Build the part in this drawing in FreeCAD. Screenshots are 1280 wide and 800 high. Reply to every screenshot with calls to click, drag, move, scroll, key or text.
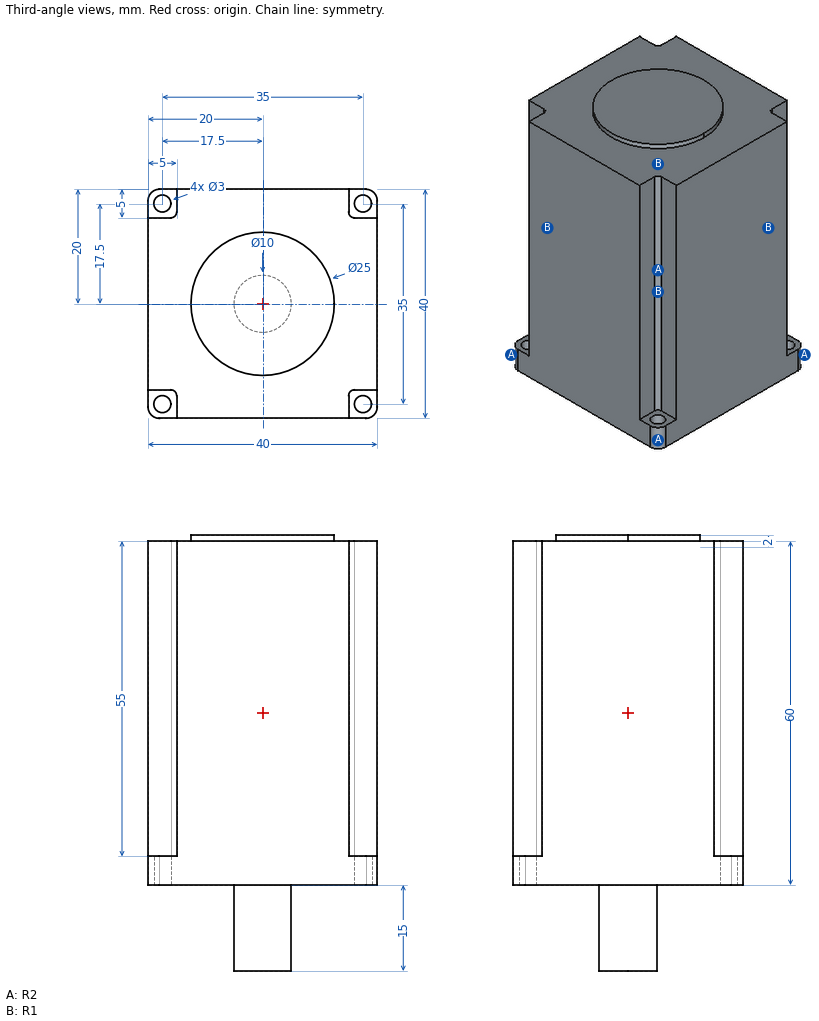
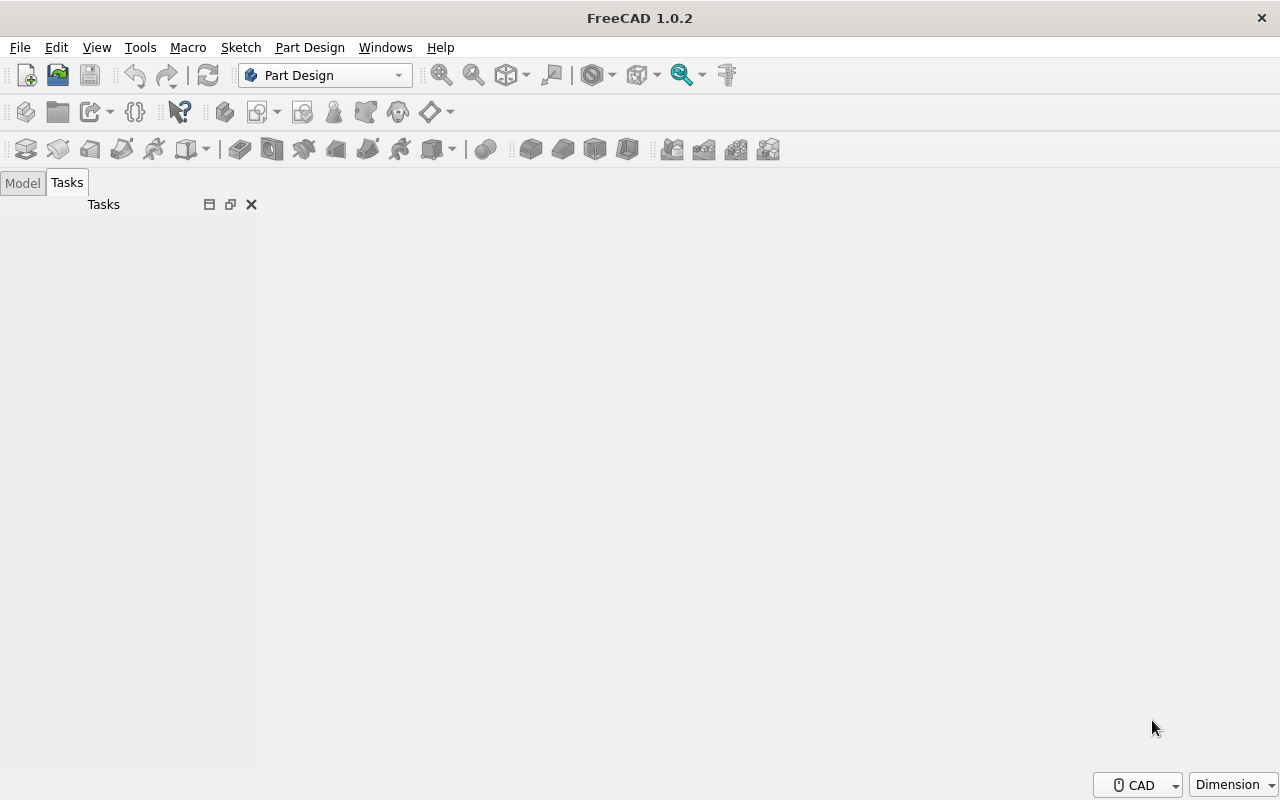
click(26, 76)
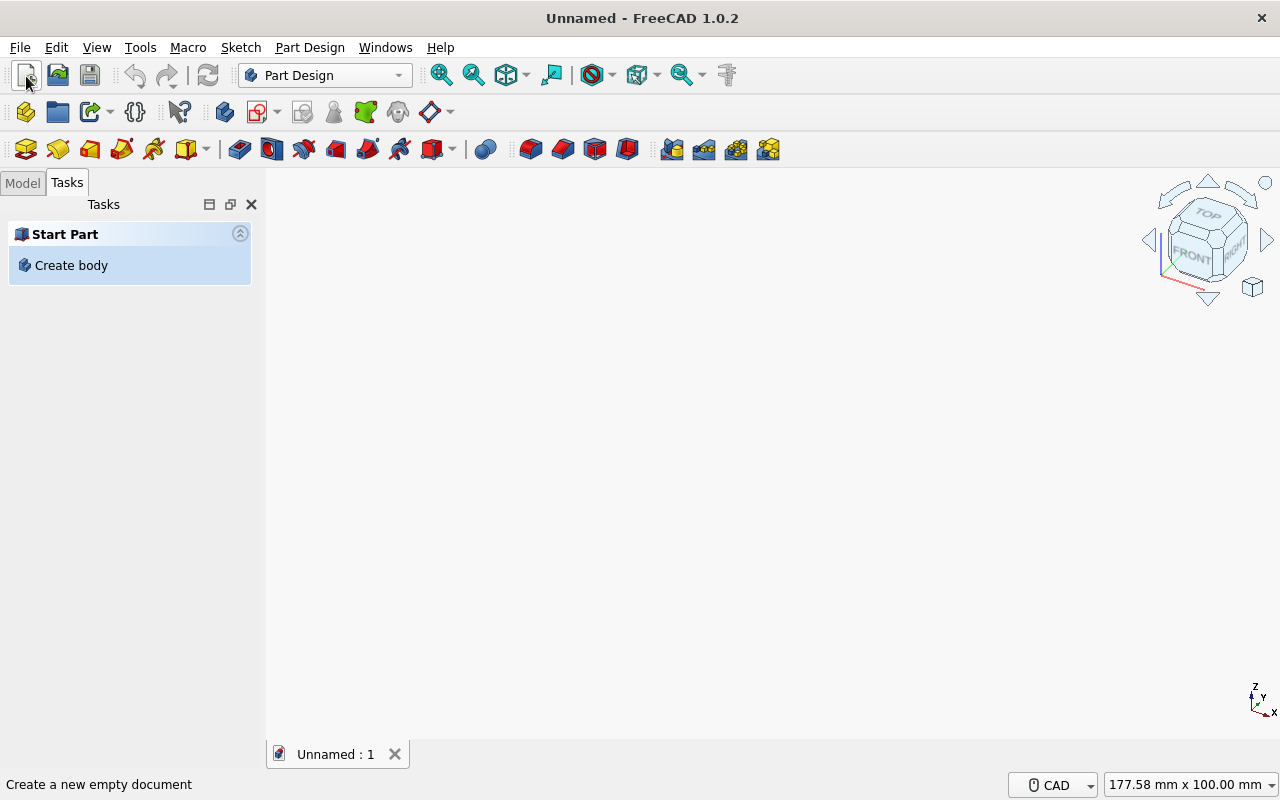
click(258, 112)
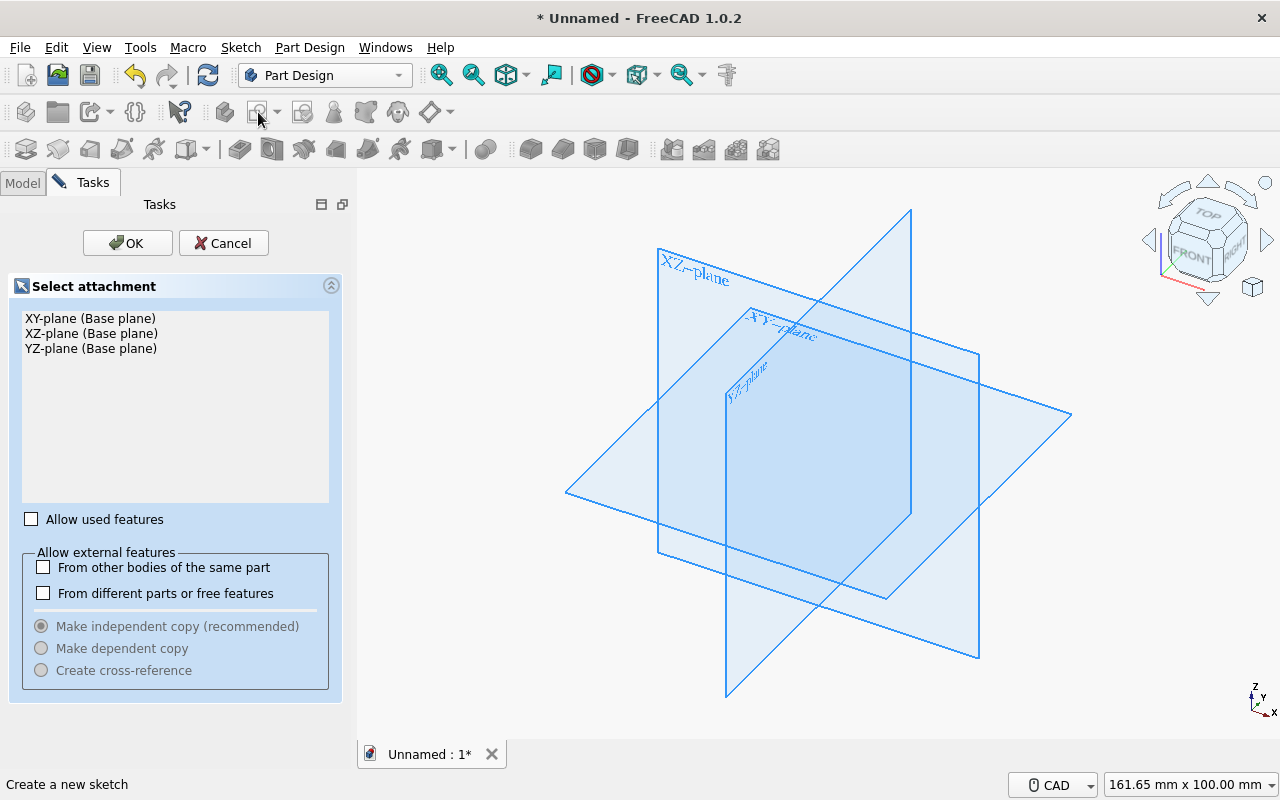
click(82, 318)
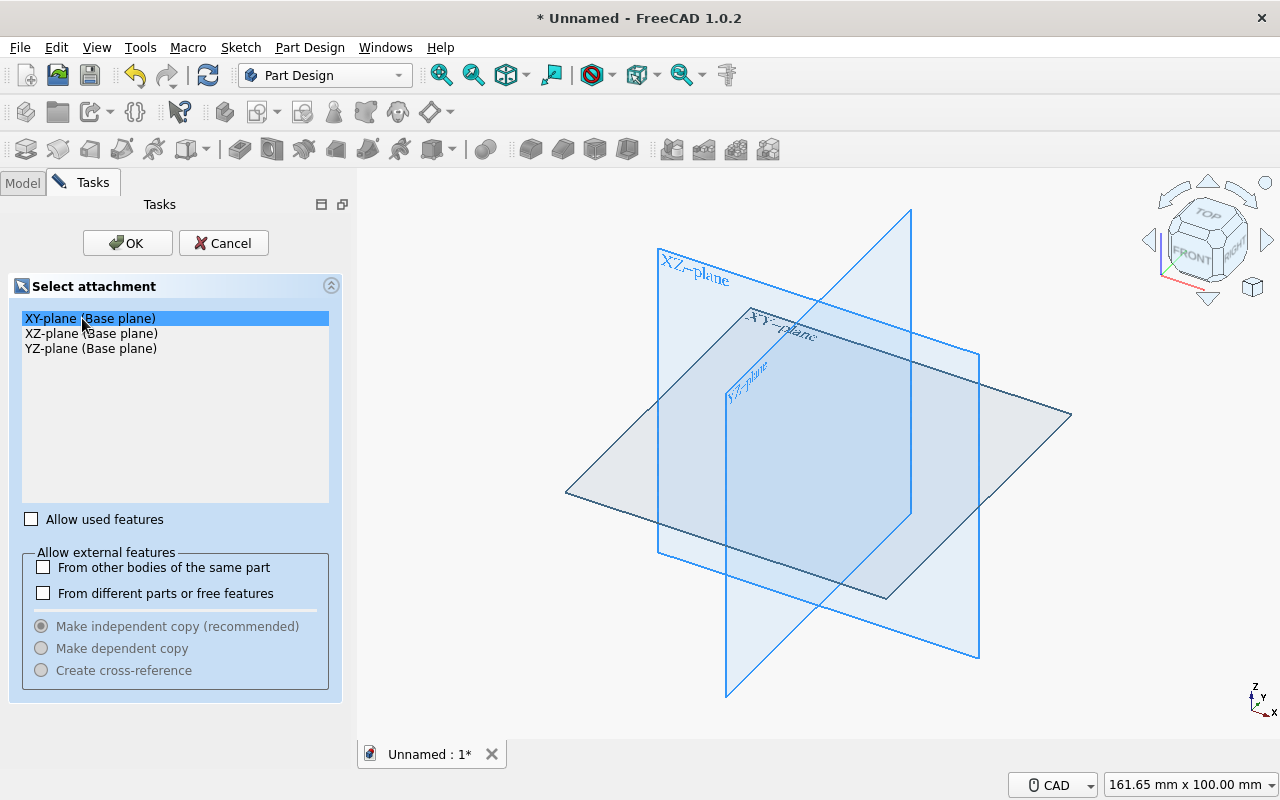
click(128, 243)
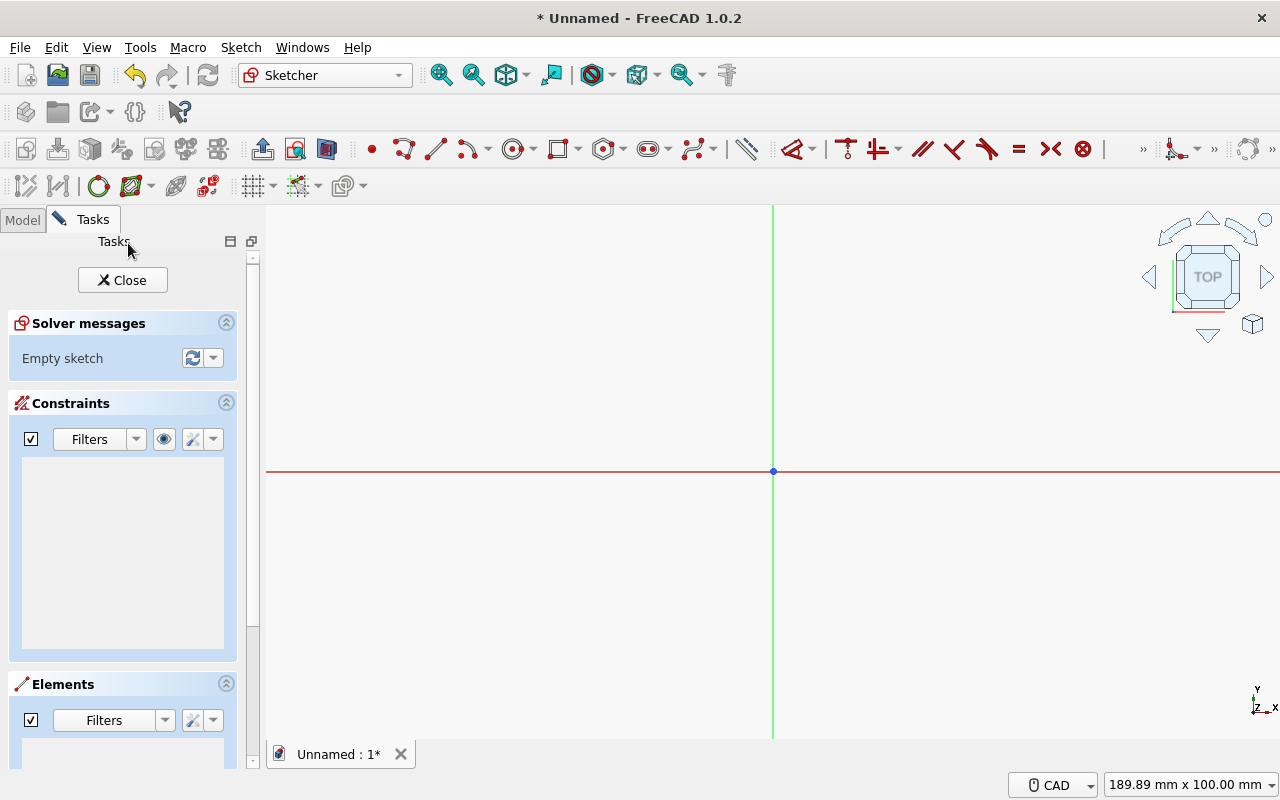
scroll(912, 472, up, 2)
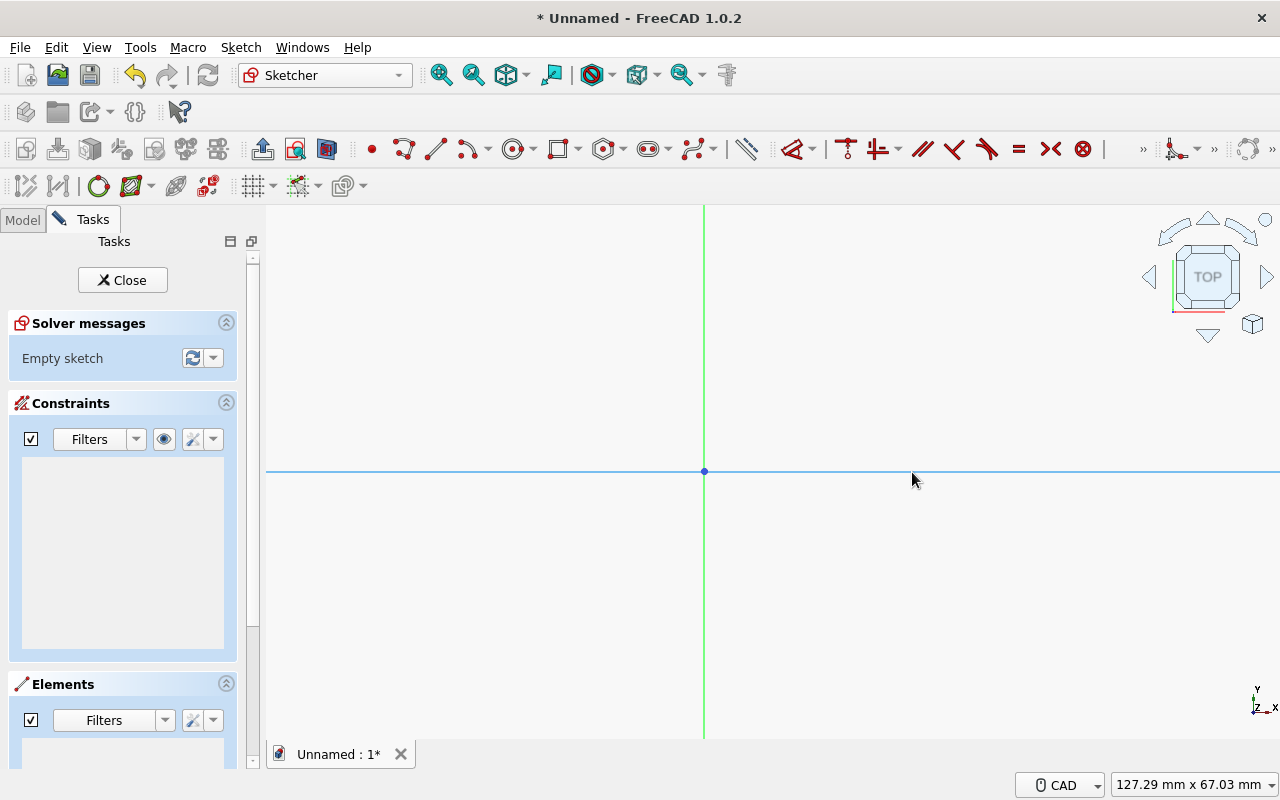
key(g)
key(v)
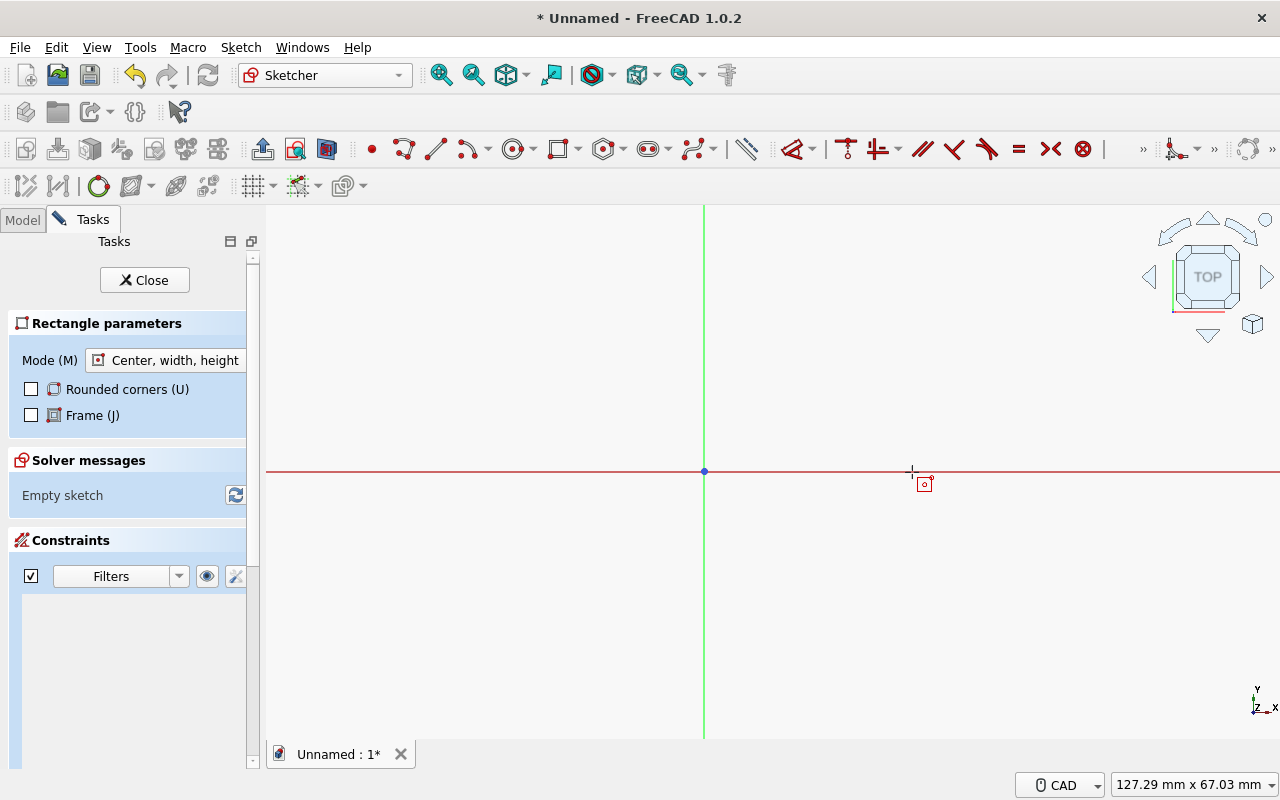
click(704, 472)
click(864, 312)
key(Escape)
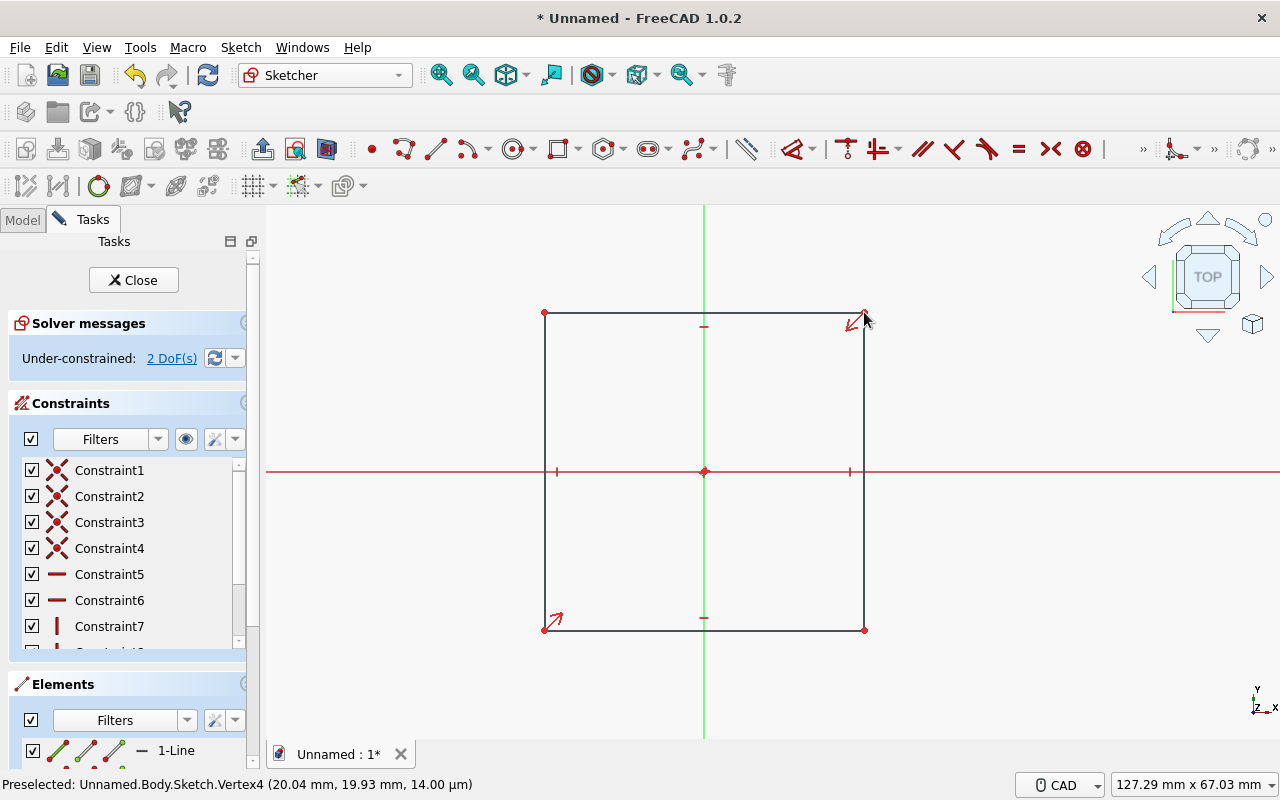
click(792, 150)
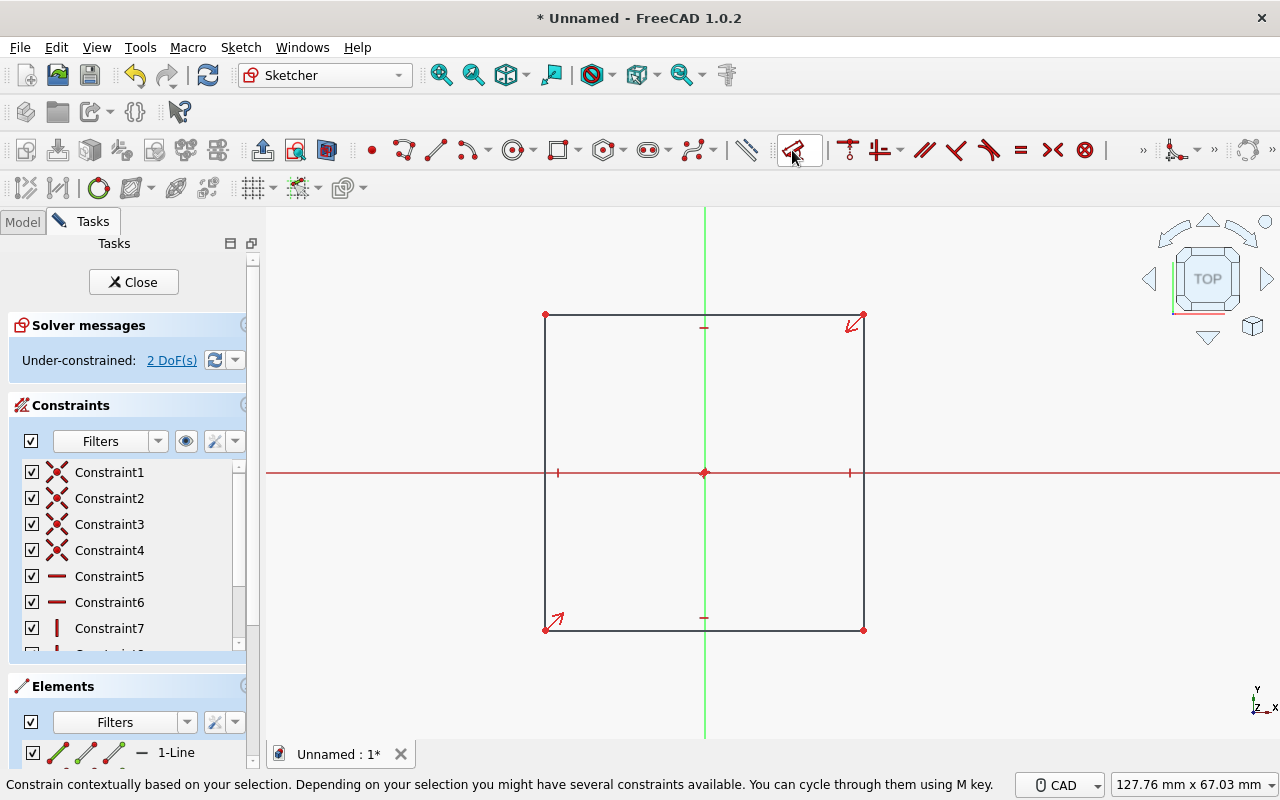
click(641, 631)
click(631, 665)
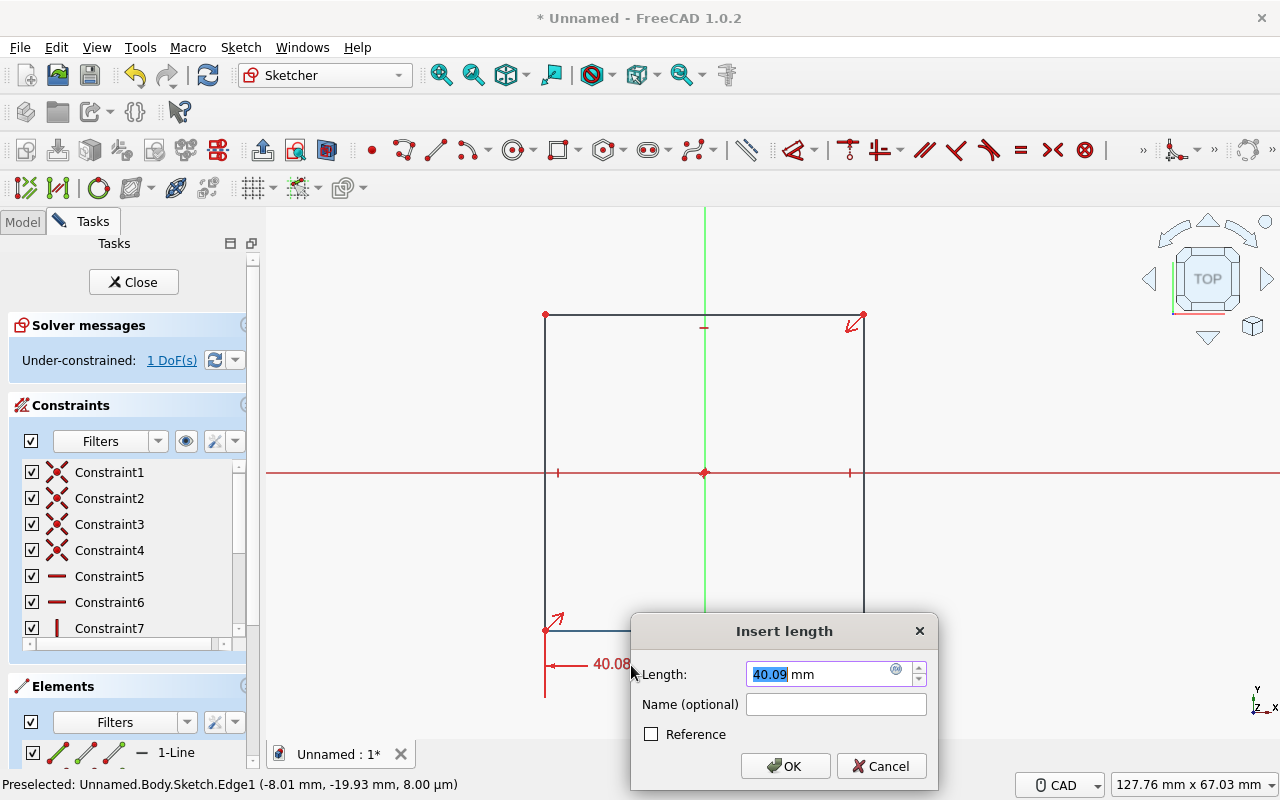
text(40)
key(Return)